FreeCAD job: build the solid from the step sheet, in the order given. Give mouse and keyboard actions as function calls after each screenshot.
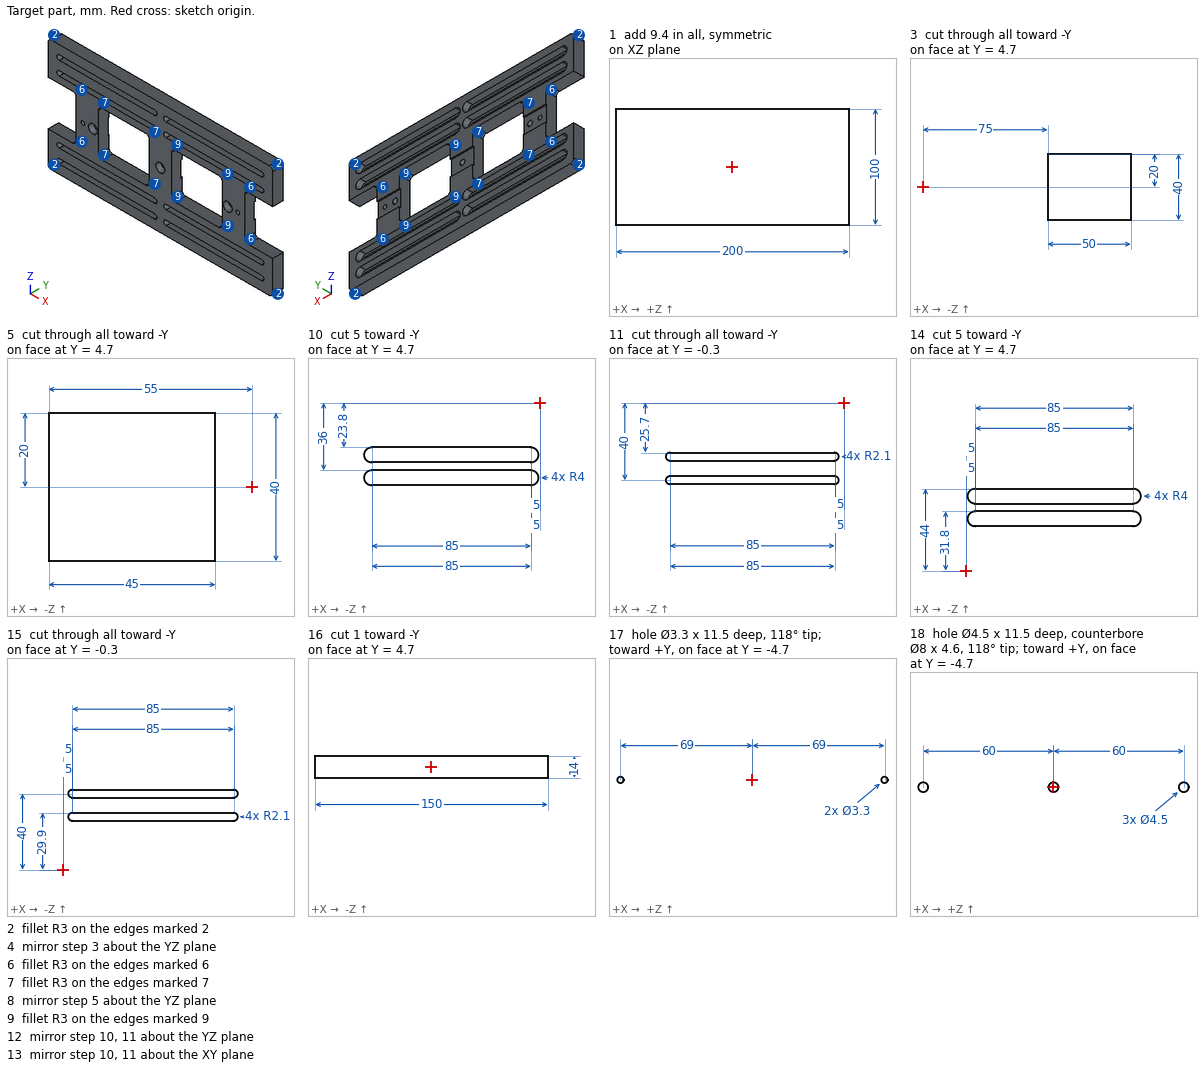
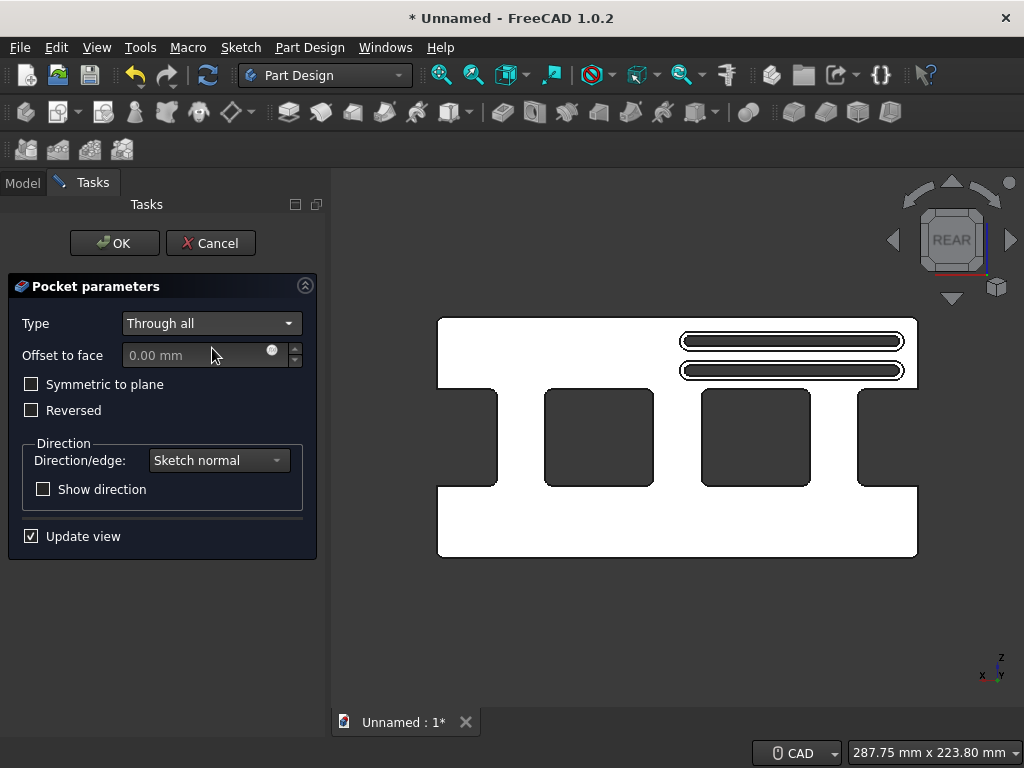
click(115, 243)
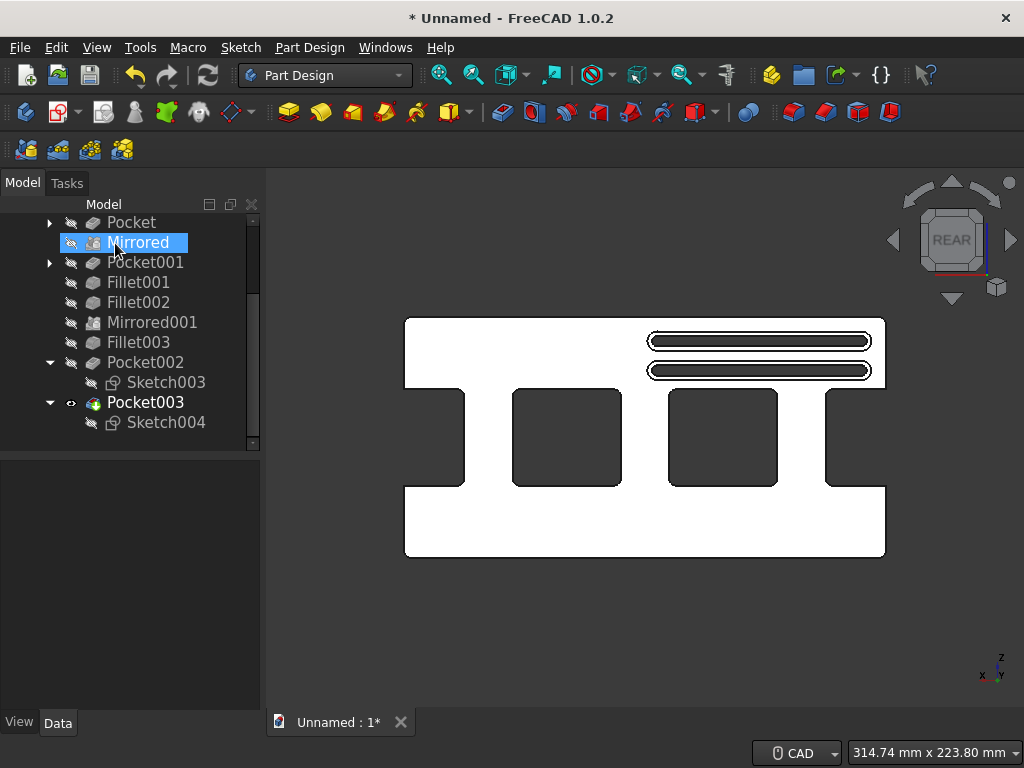
click(116, 363)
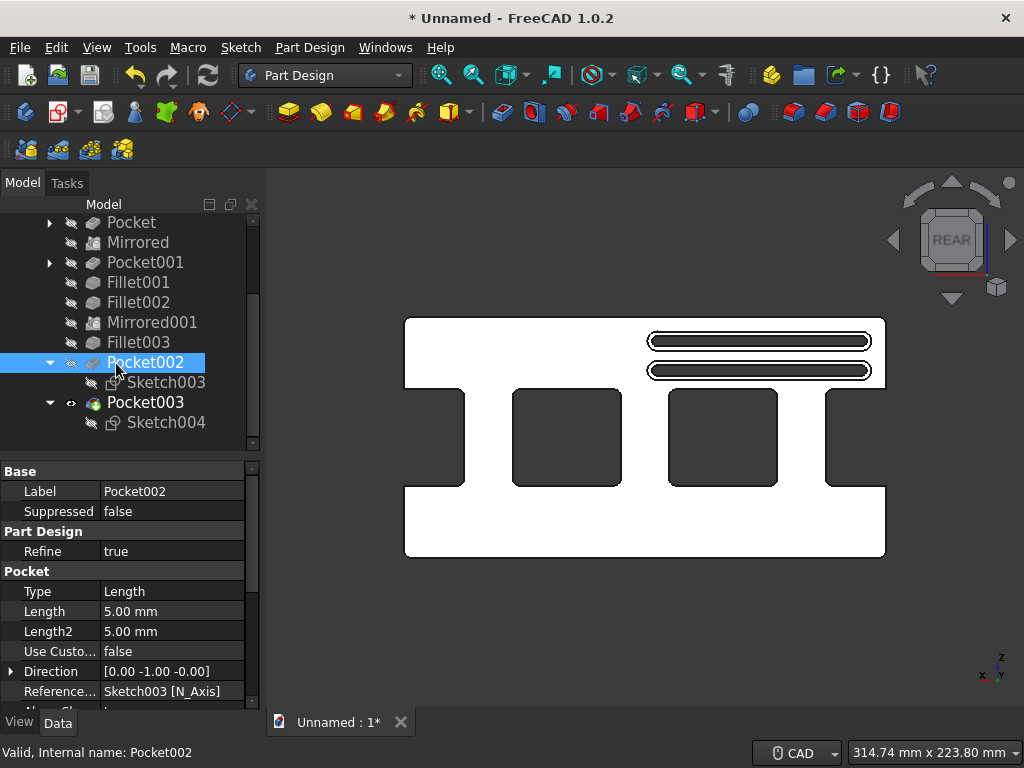
click(116, 403, ctrl)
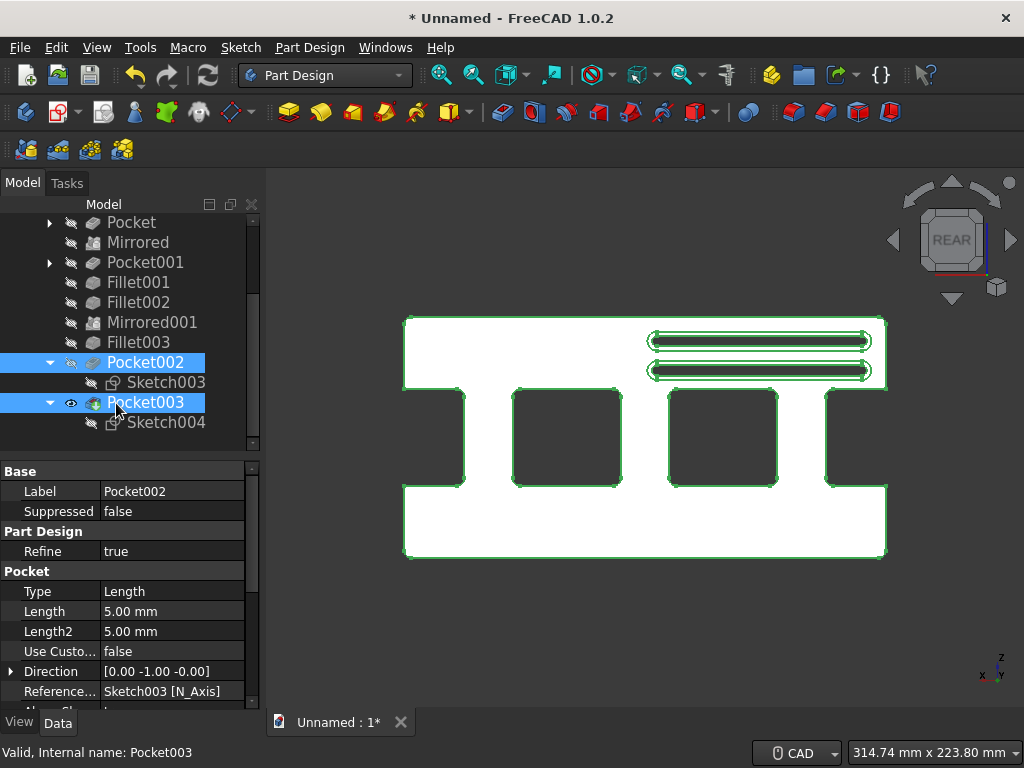
click(26, 150)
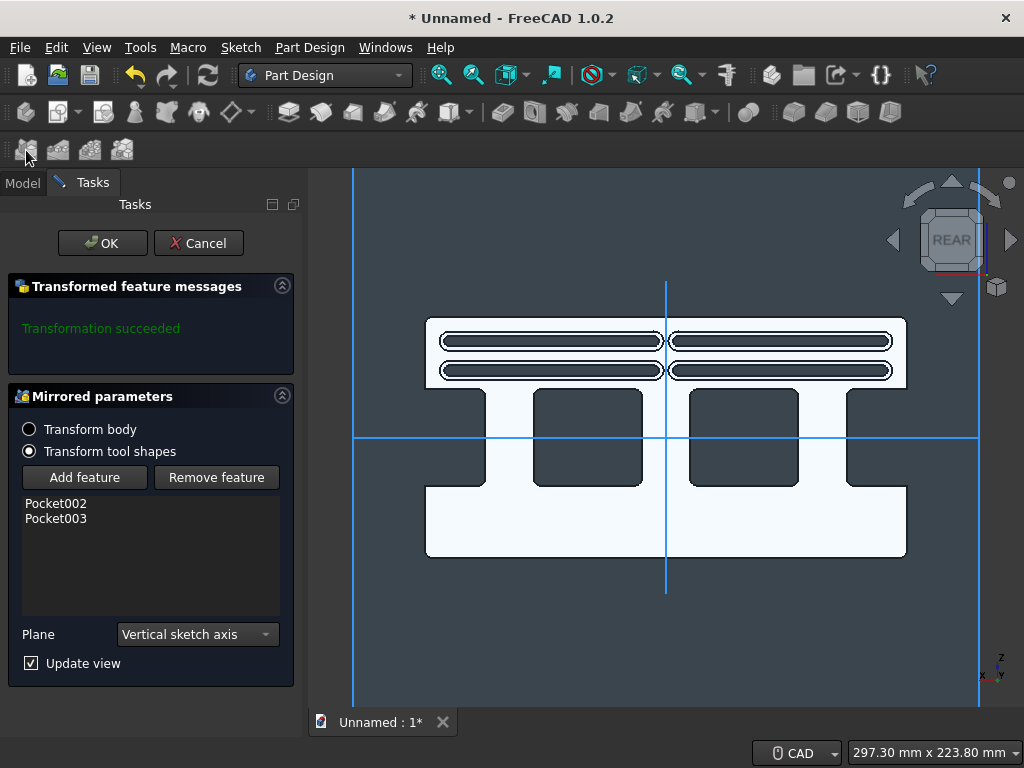
click(198, 634)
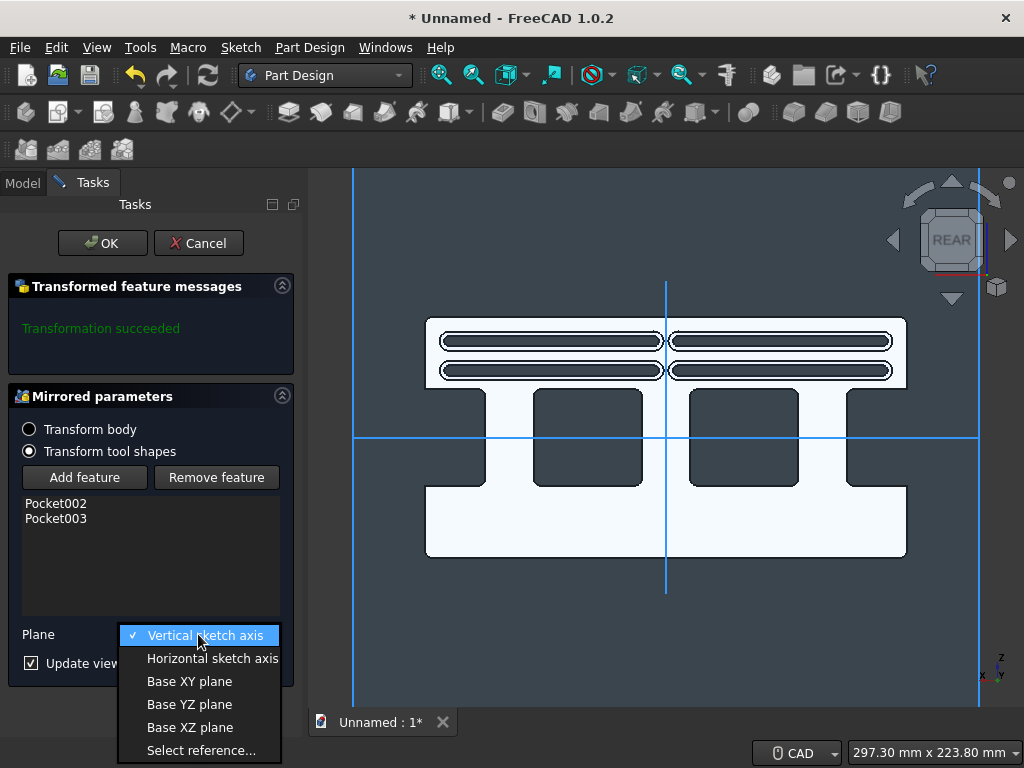
click(198, 704)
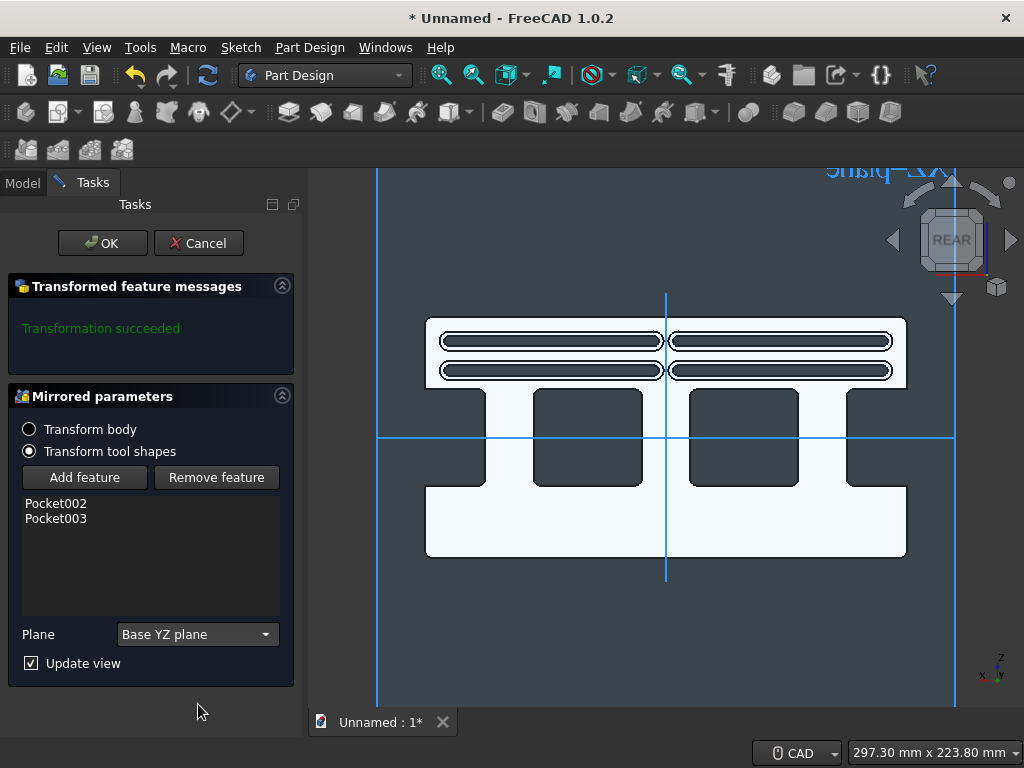
click(103, 243)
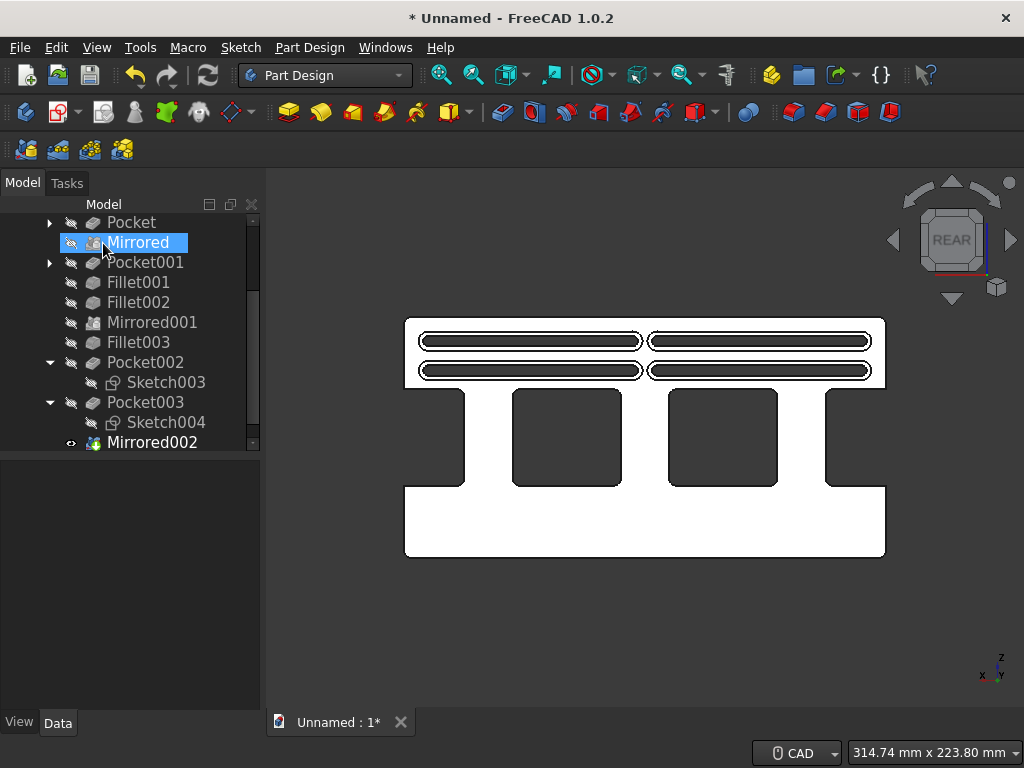
click(116, 363)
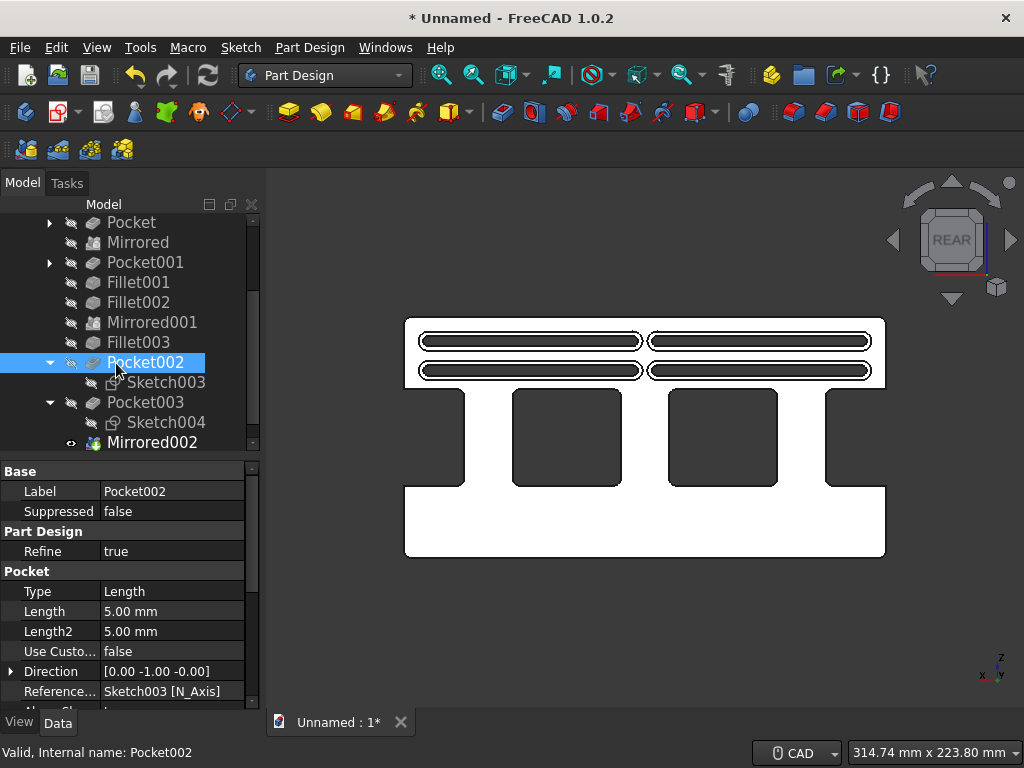
click(116, 403, ctrl)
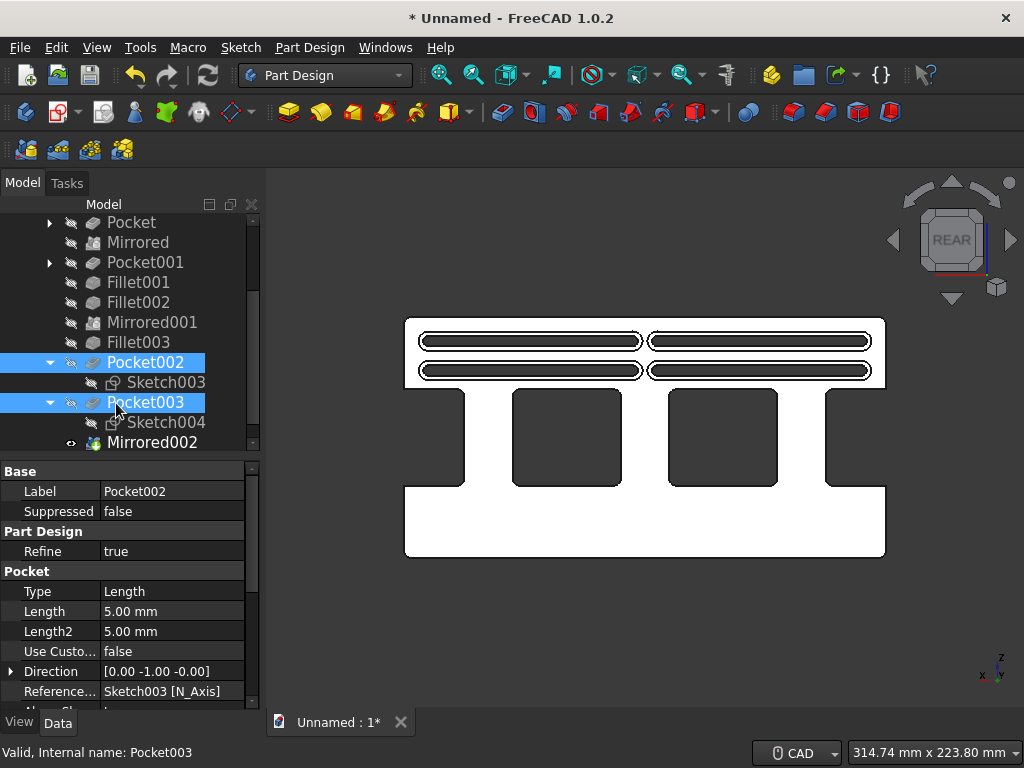
click(26, 150)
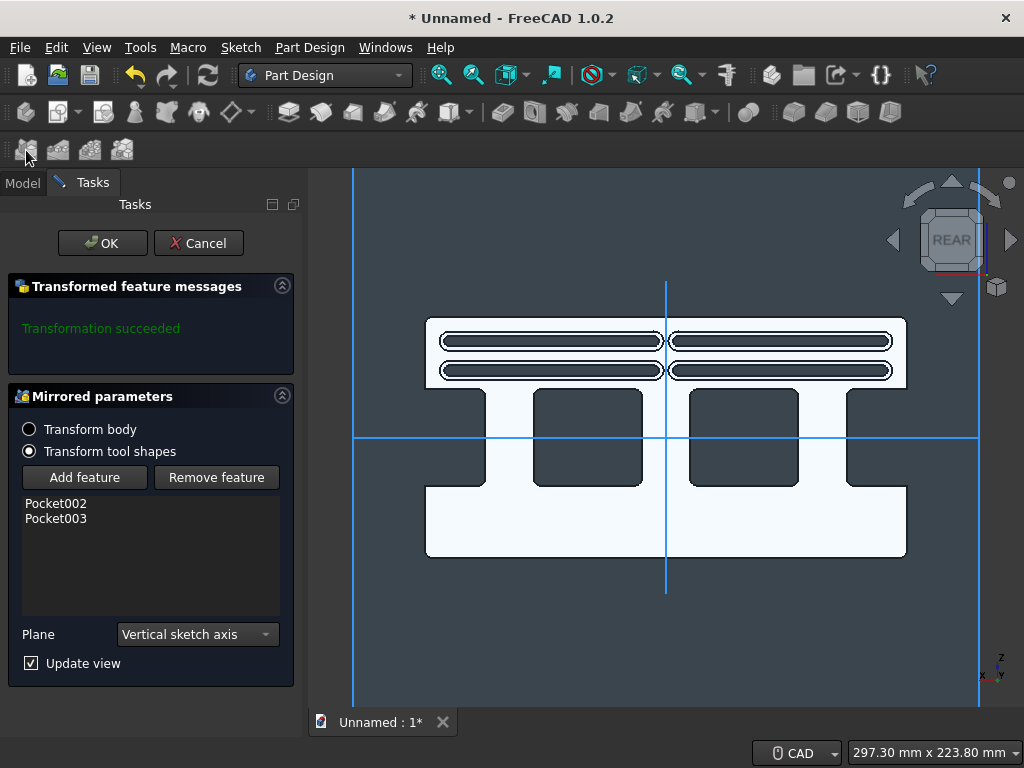
click(198, 634)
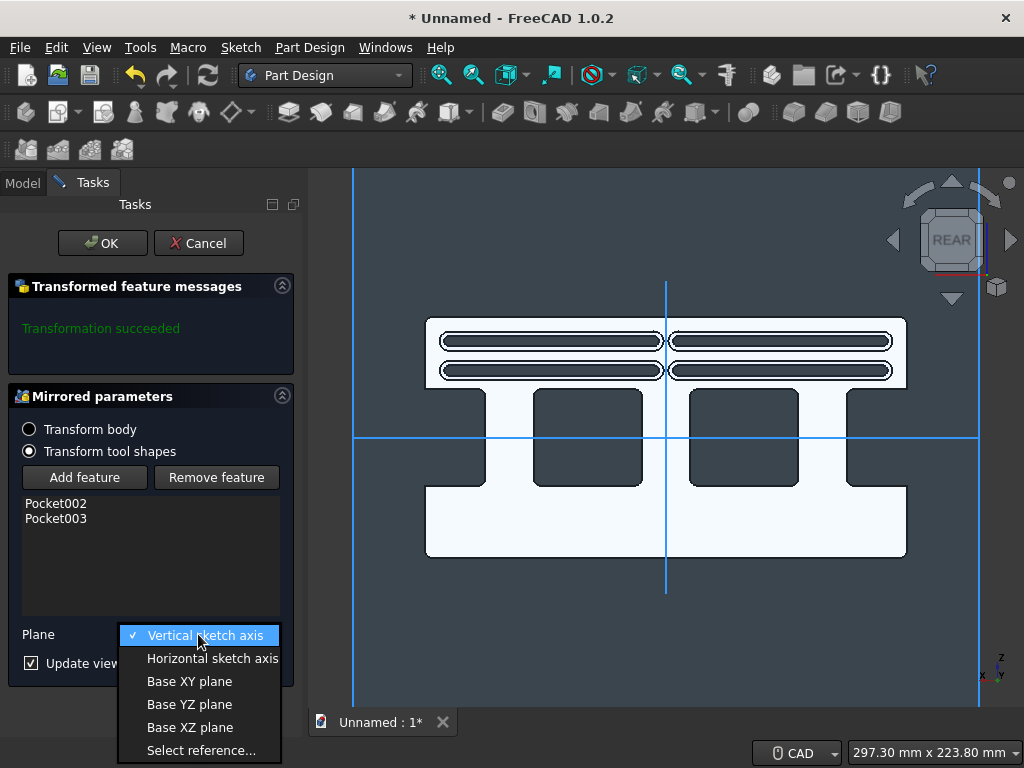
click(198, 682)